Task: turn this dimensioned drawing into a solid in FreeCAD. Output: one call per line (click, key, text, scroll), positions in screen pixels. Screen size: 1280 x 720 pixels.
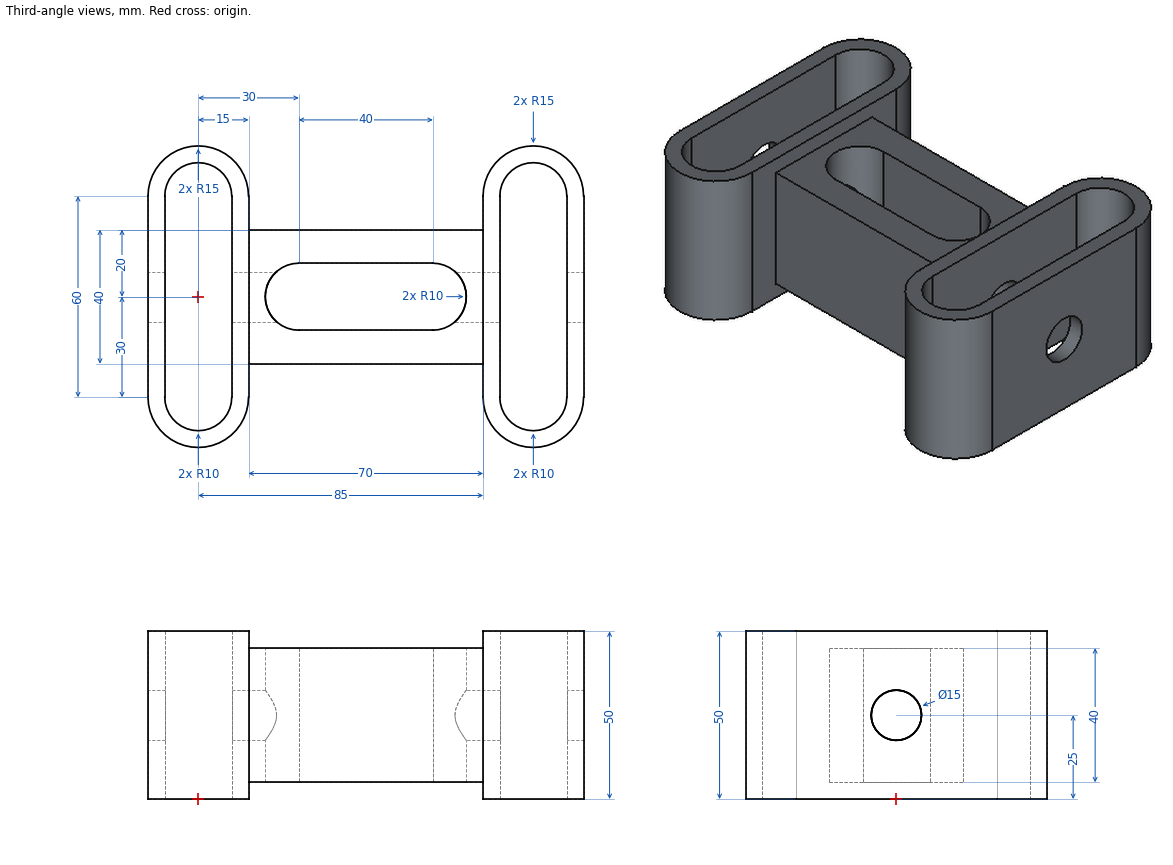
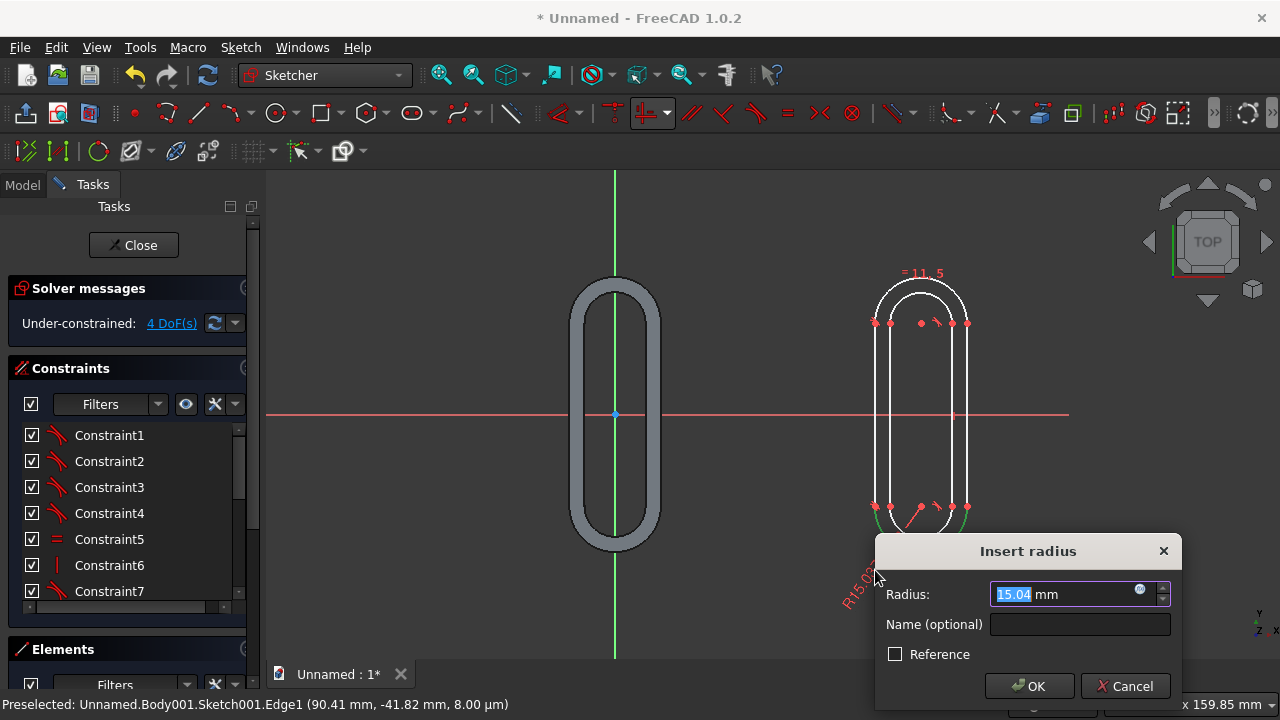
text(15)
key(Return)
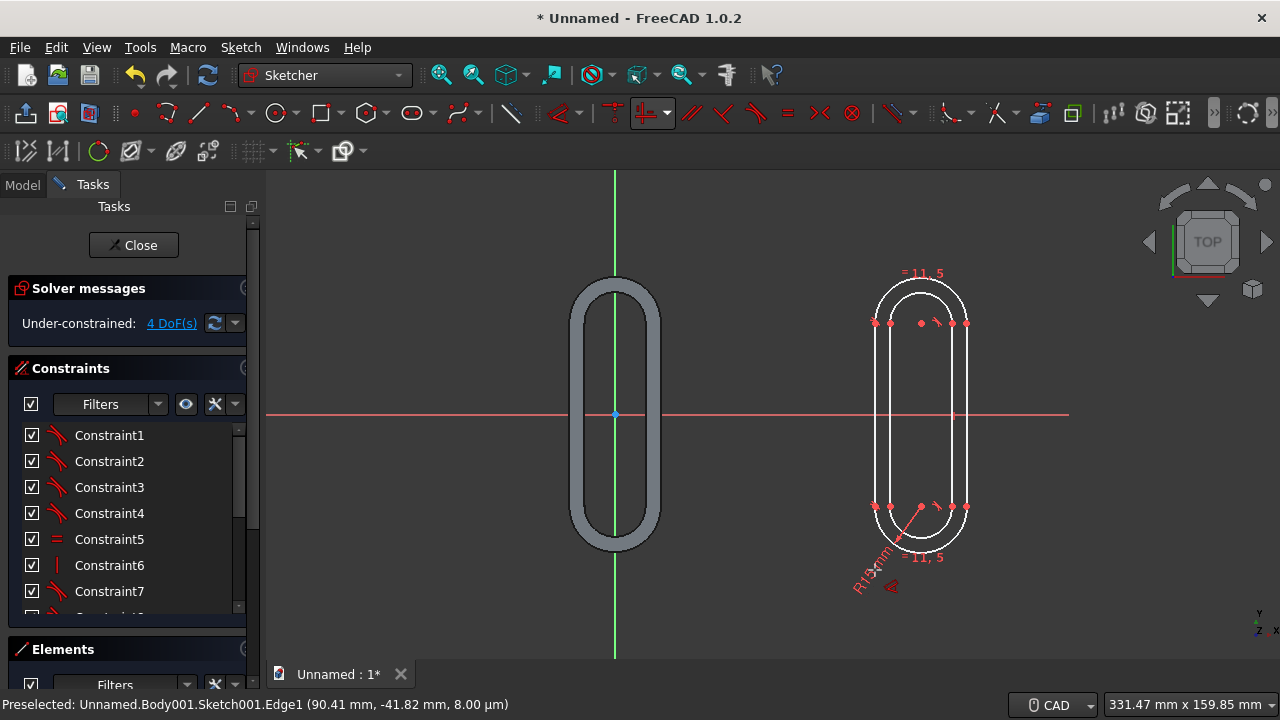
scroll(903, 532, up, 2)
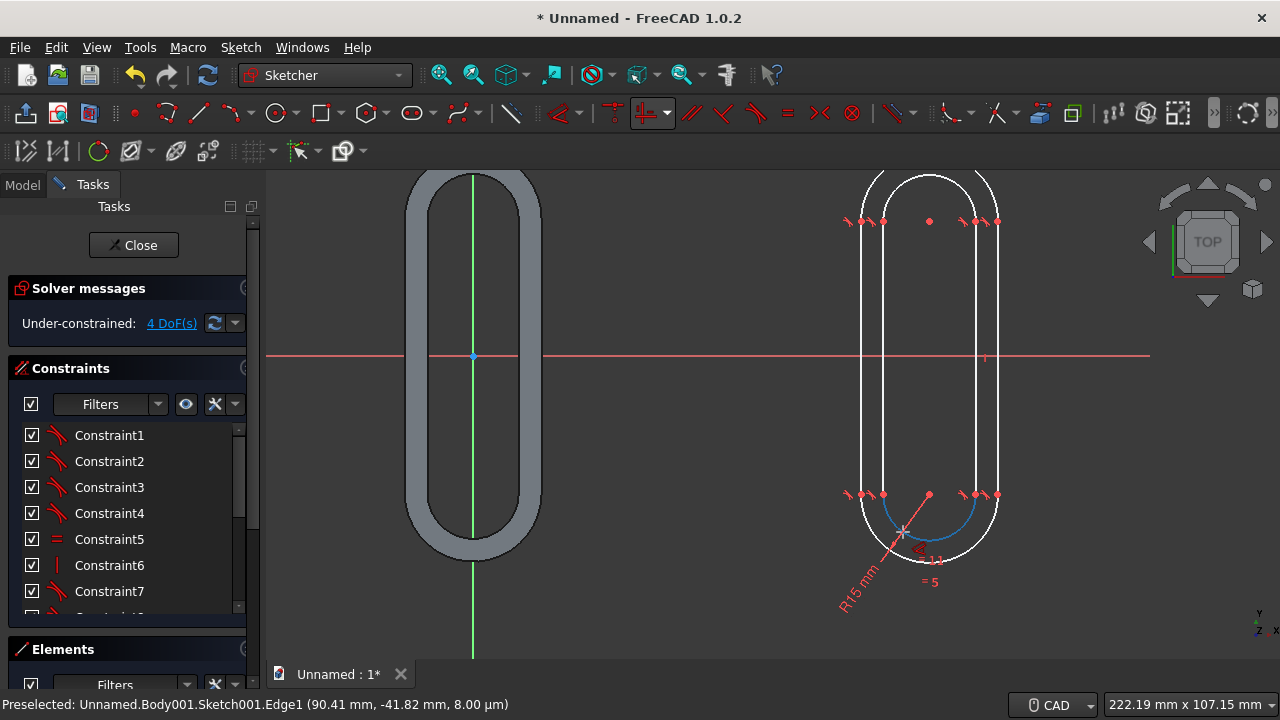
click(902, 532)
click(838, 538)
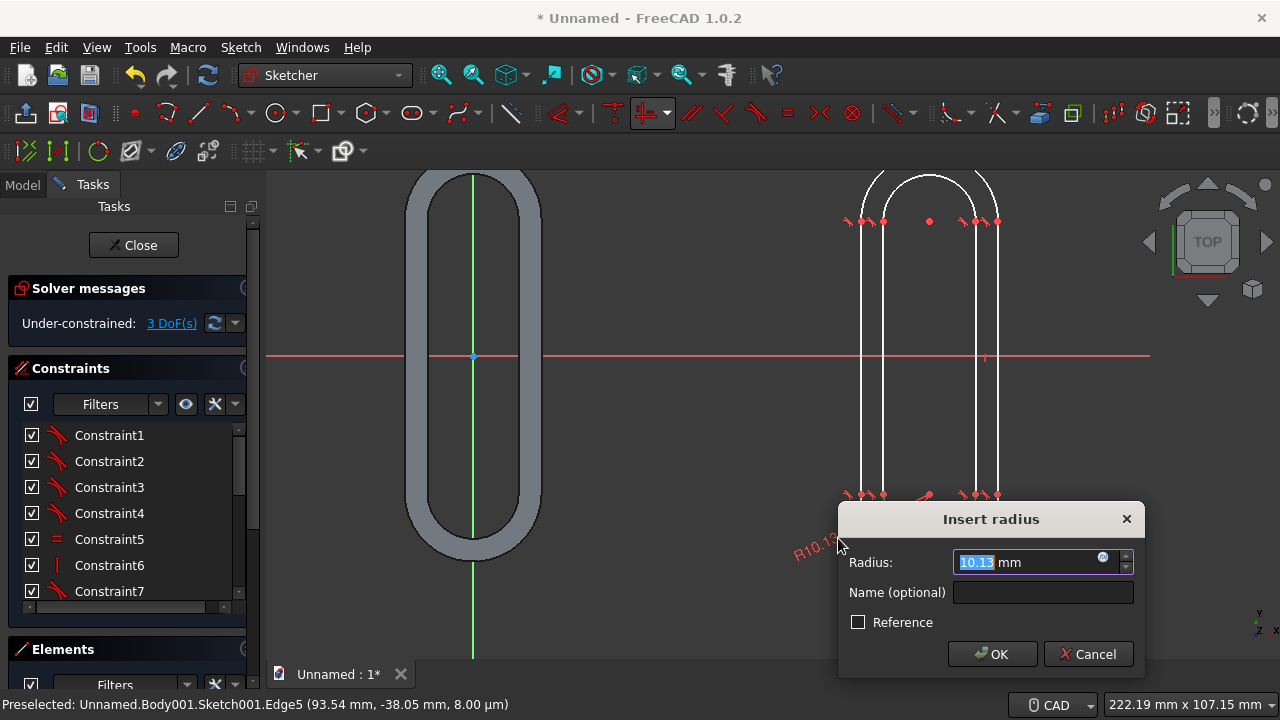
text(10)
key(Return)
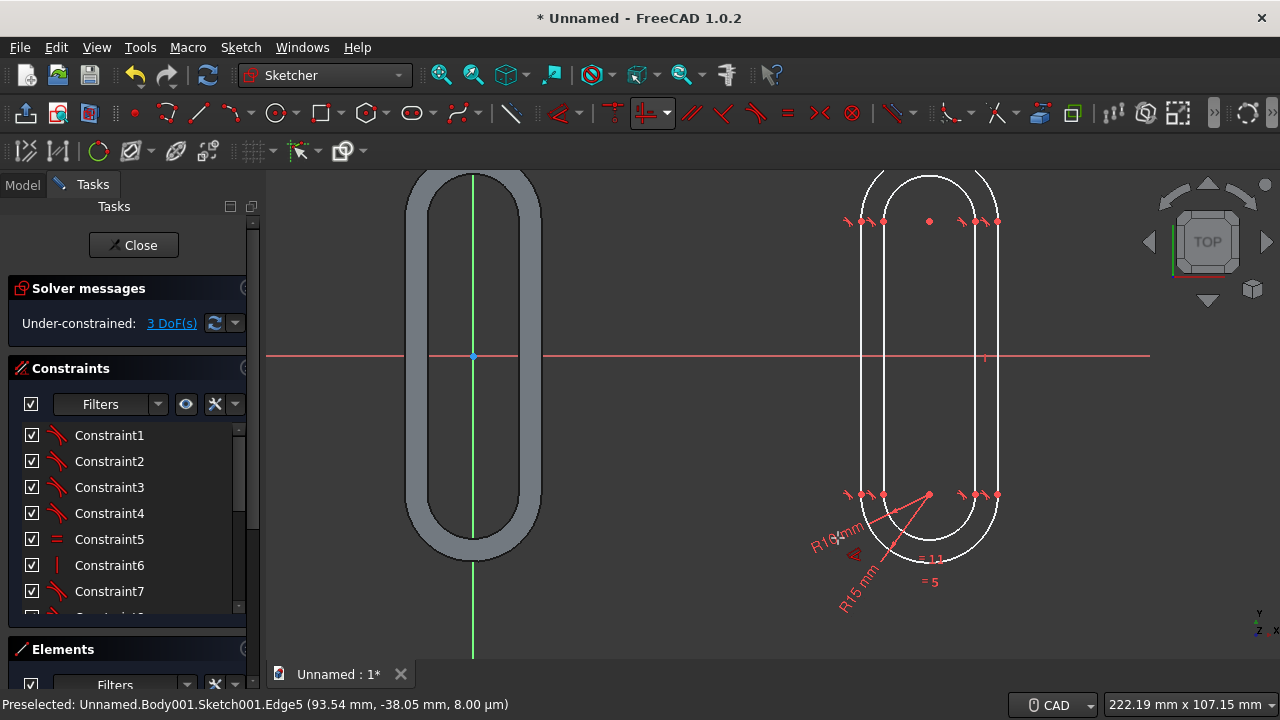
click(861, 412)
click(827, 295)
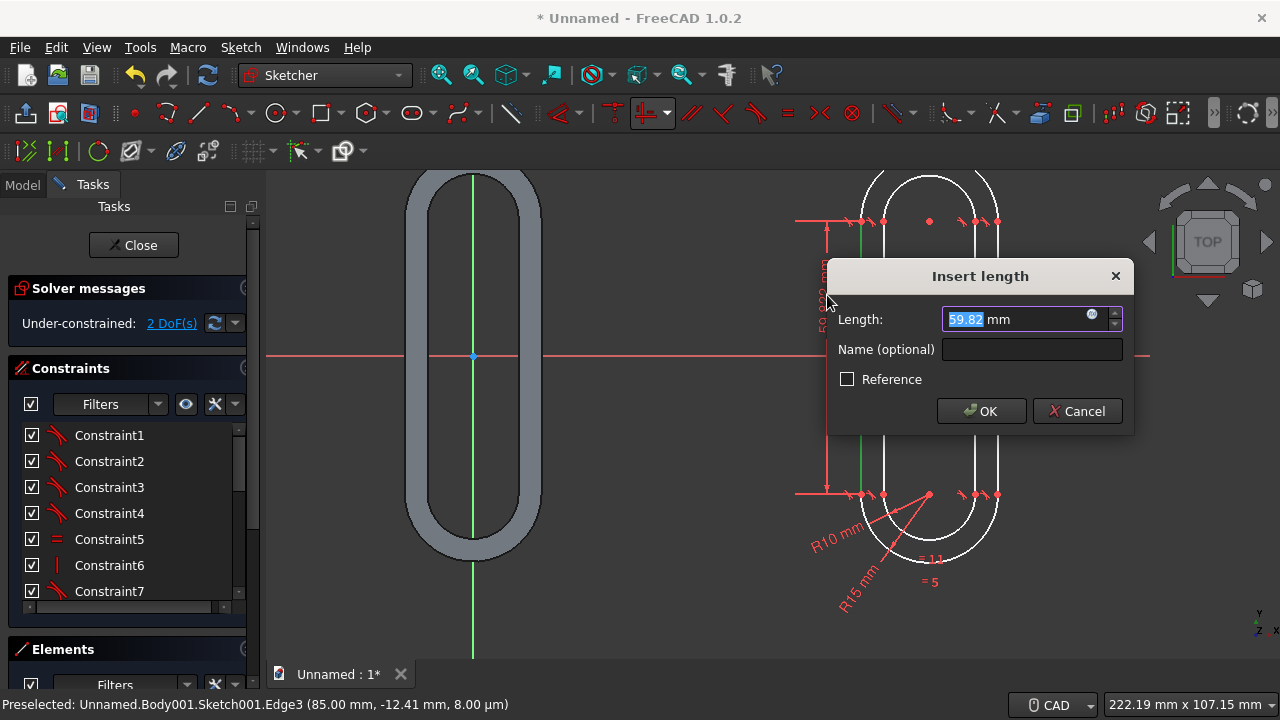
text(60)
key(Return)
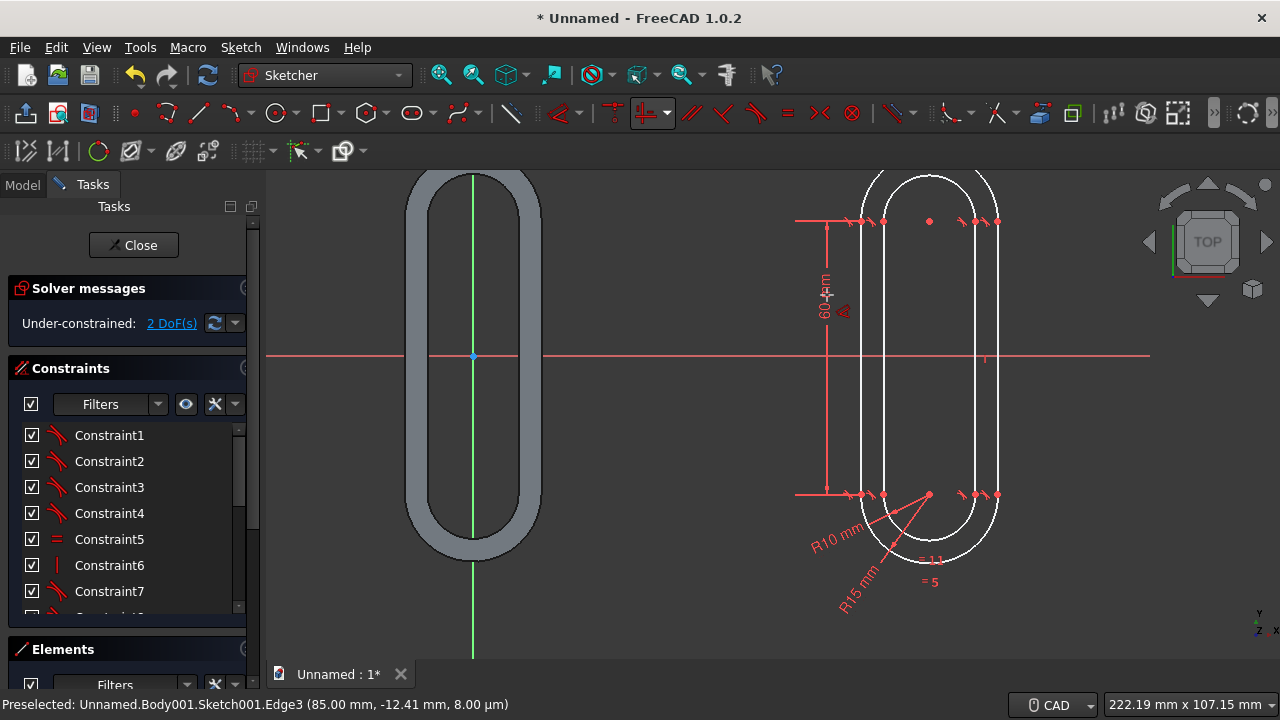
click(861, 495)
click(667, 529)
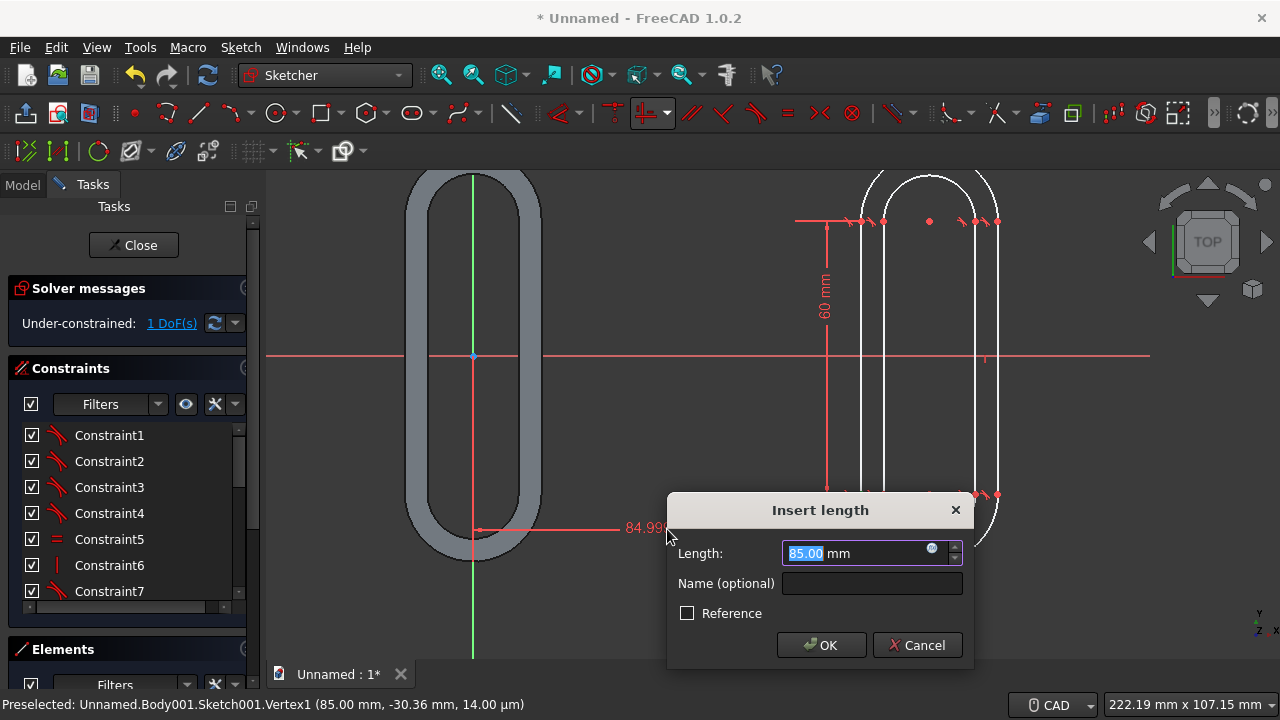
text(85)
key(Return)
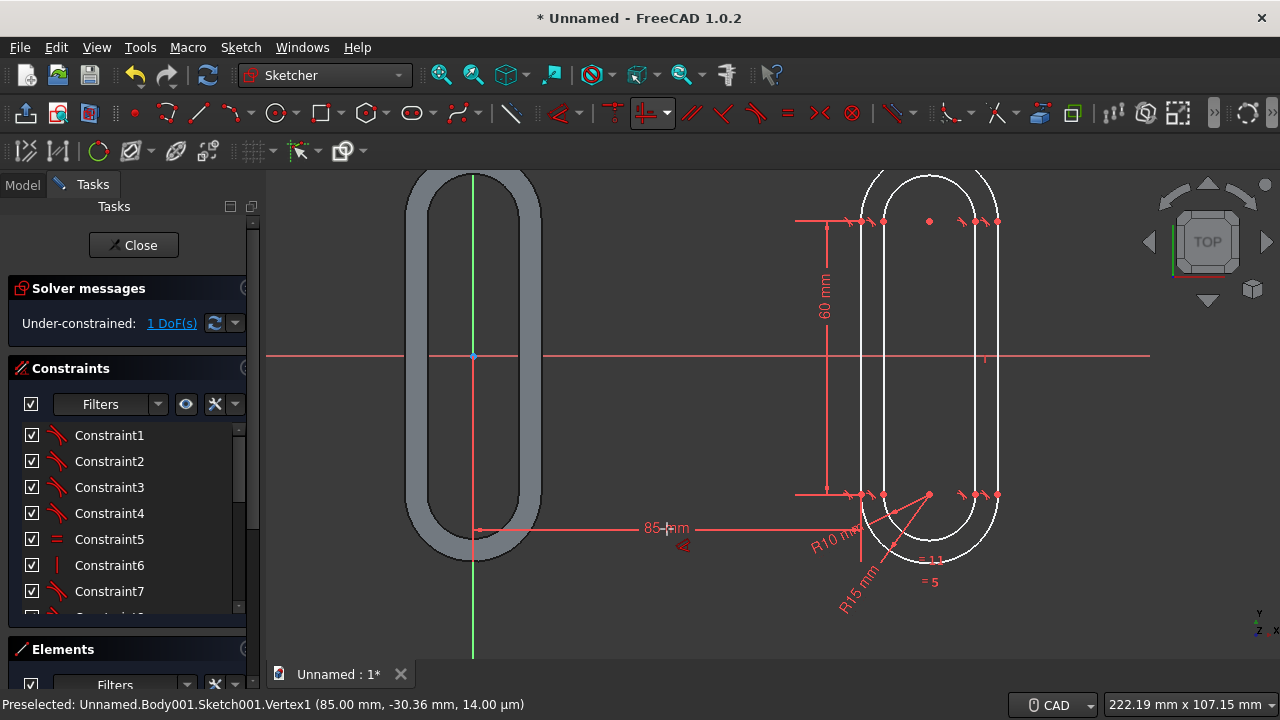
click(861, 495)
click(439, 426)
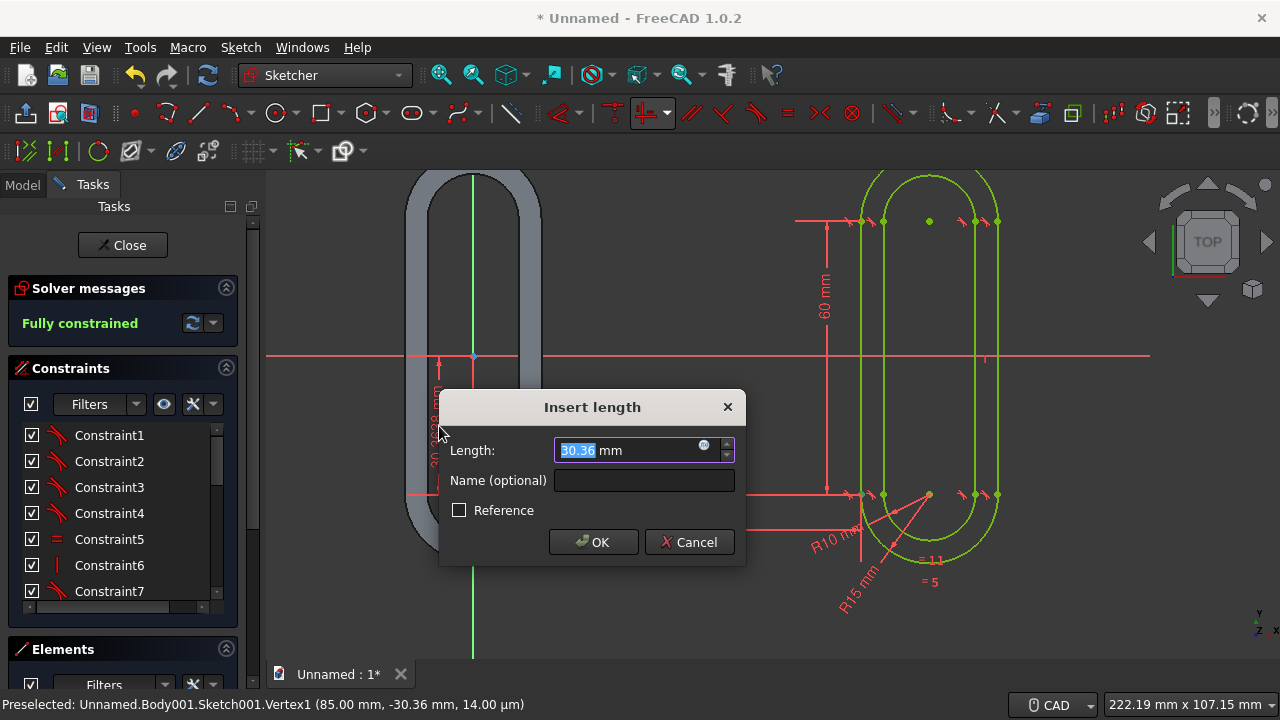
text(30)
key(Return)
key(Escape)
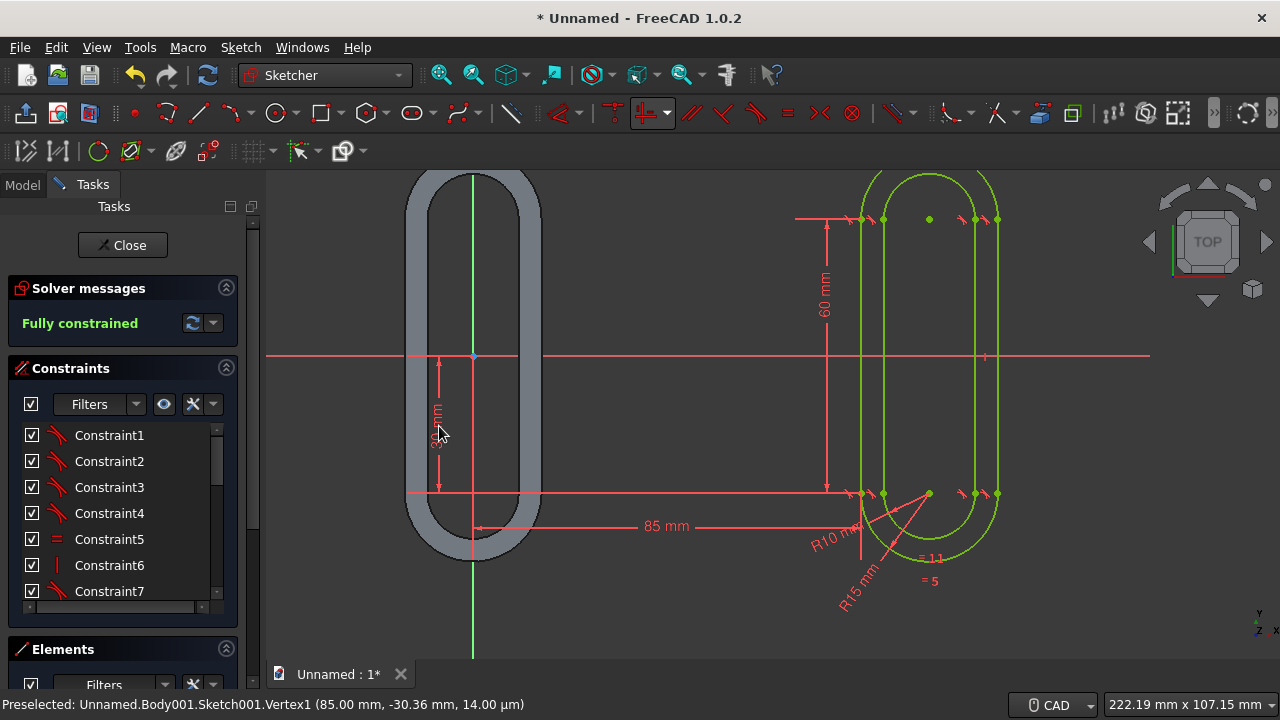
click(123, 245)